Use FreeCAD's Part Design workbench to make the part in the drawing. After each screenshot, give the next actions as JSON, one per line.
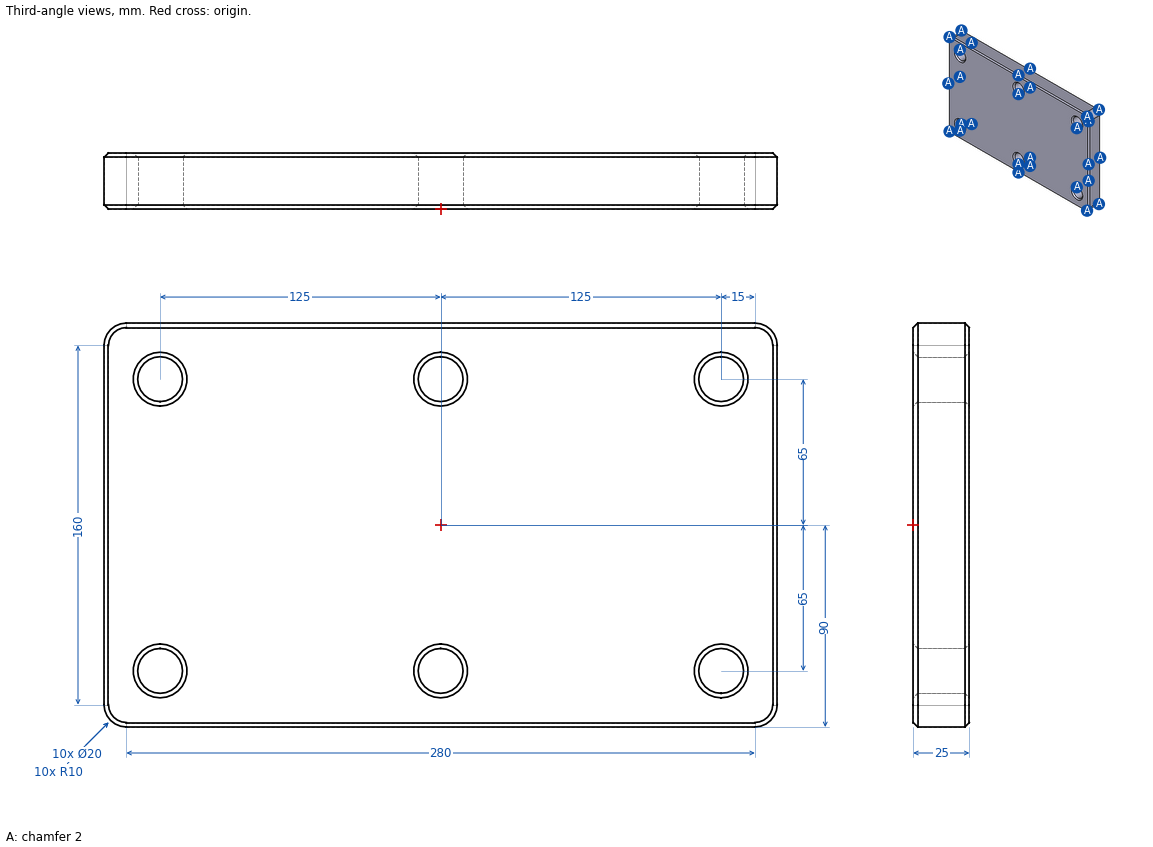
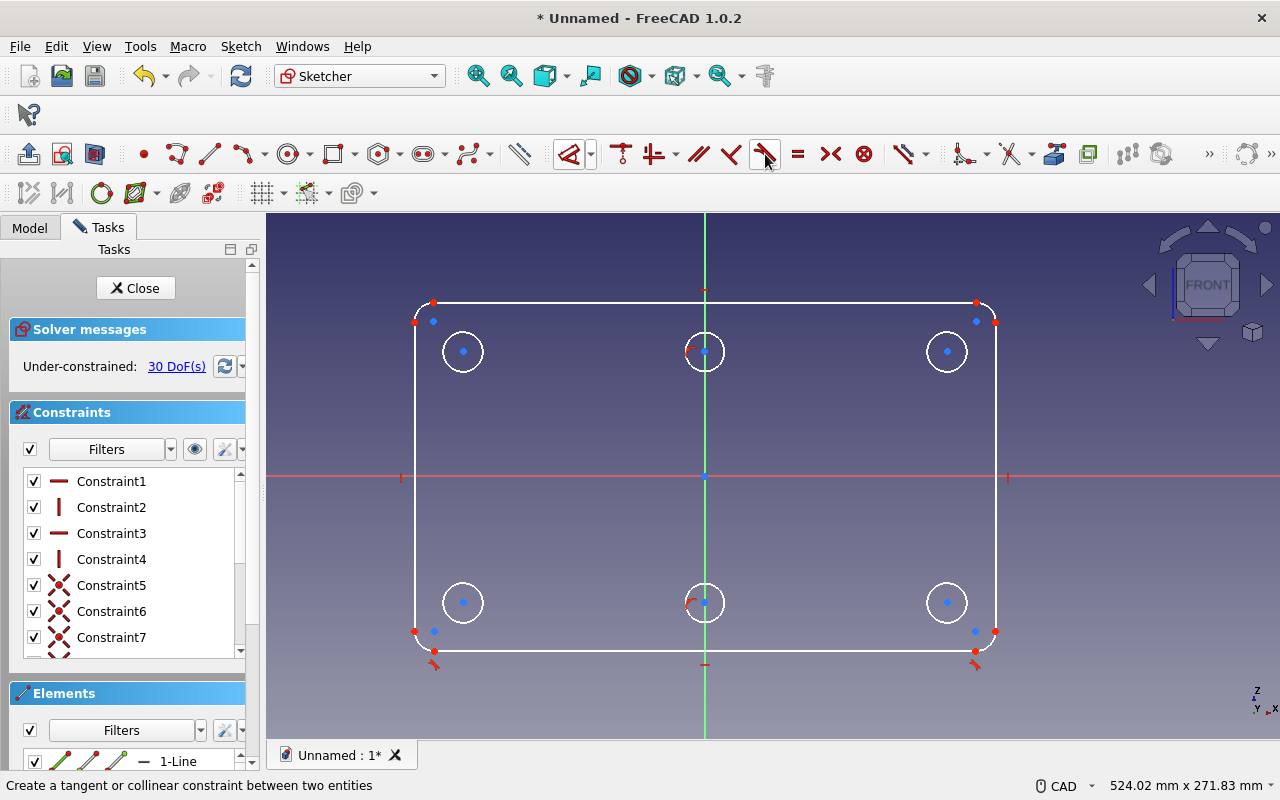
{"action": "left_click", "coordinate": [415, 539]}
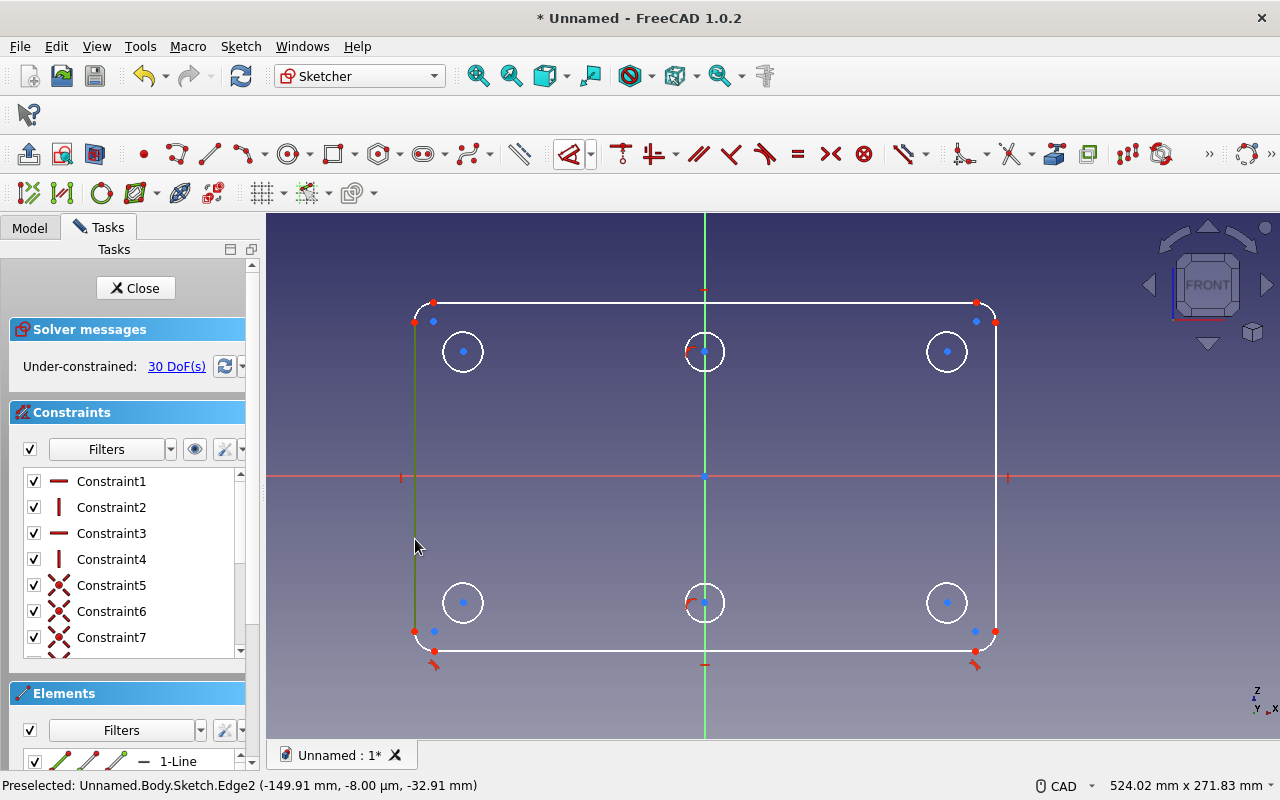
{"action": "left_click", "coordinate": [421, 645]}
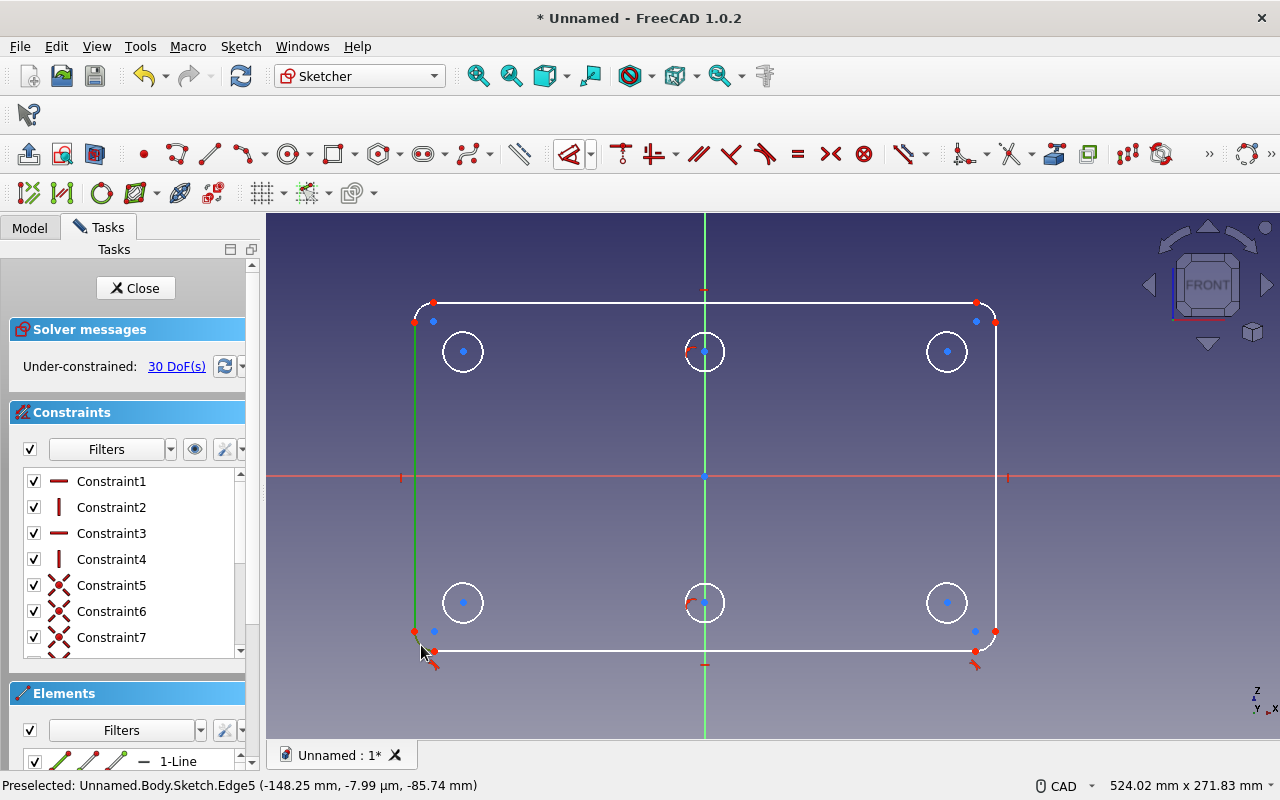
{"action": "left_click", "coordinate": [765, 154]}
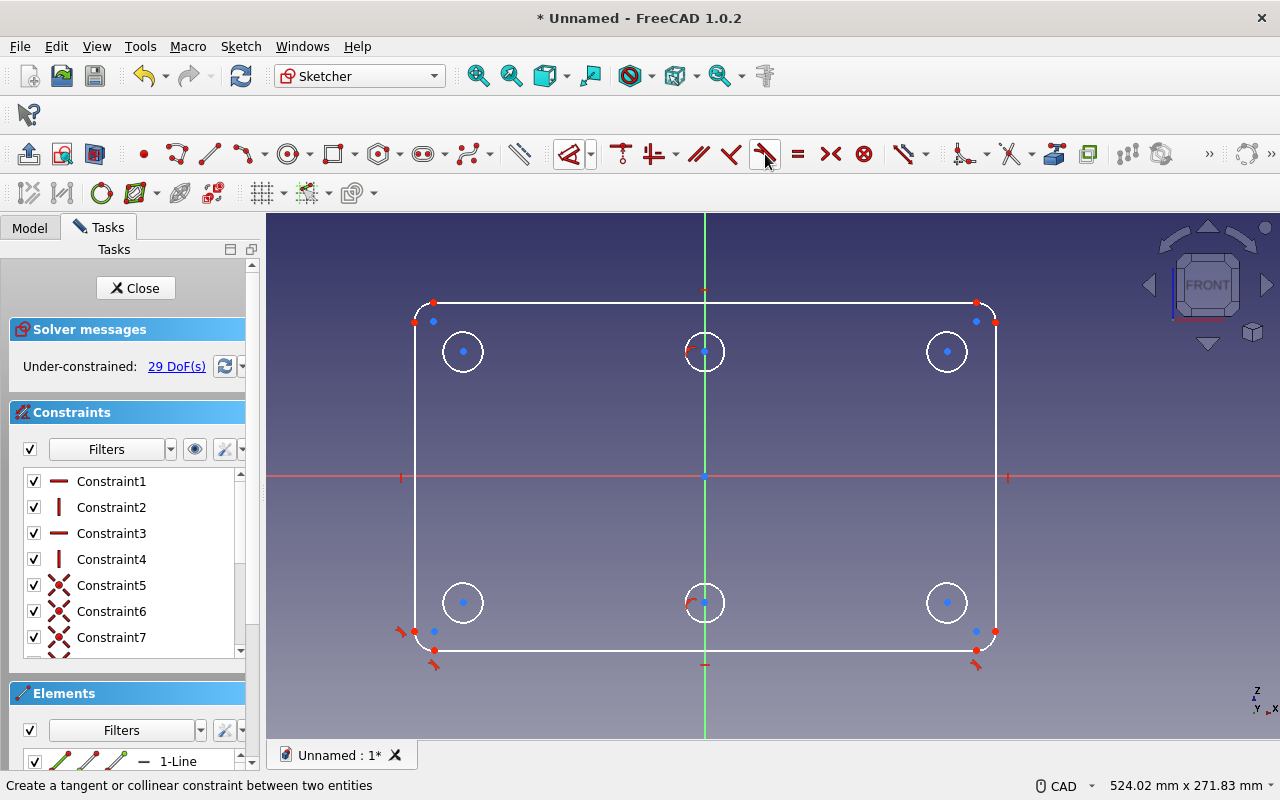
{"action": "left_click", "coordinate": [415, 539]}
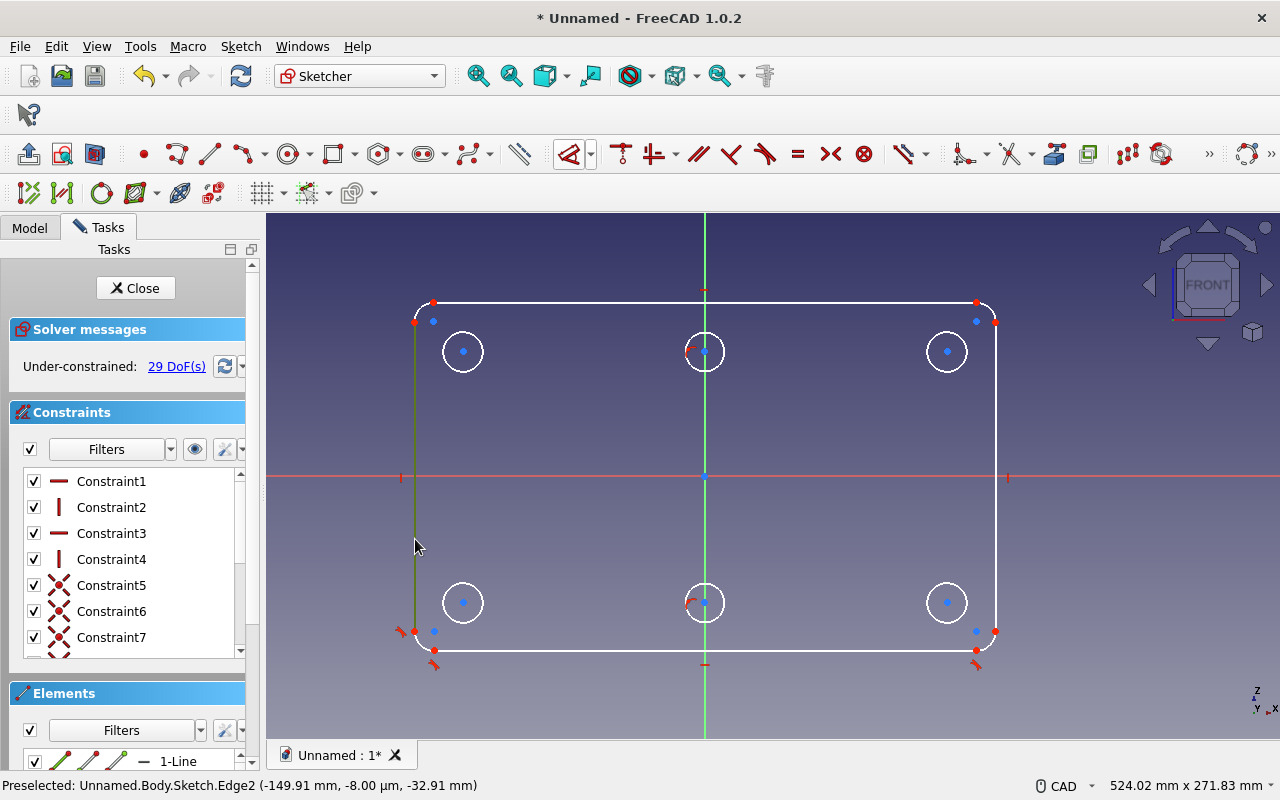
{"action": "scroll", "coordinate": [425, 305], "scroll_direction": "up", "scroll_amount": 2}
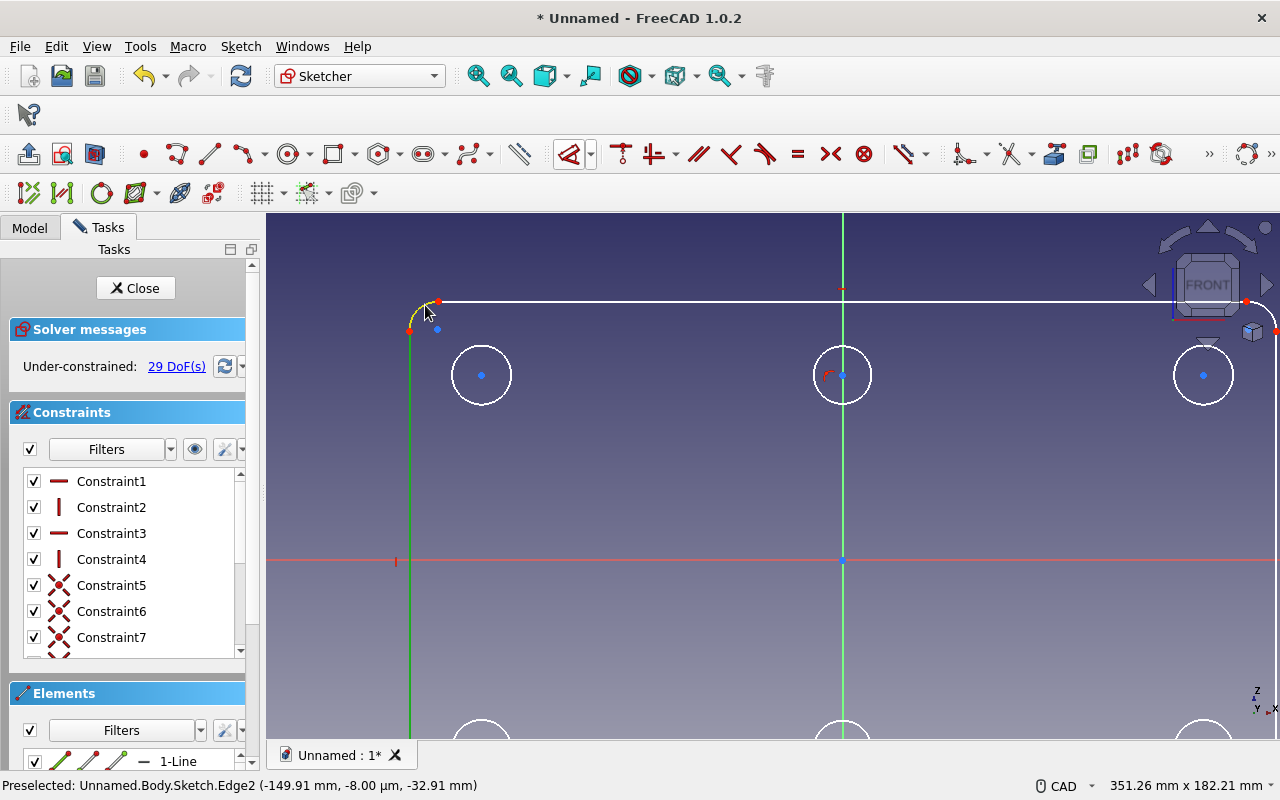
{"action": "left_click", "coordinate": [425, 305]}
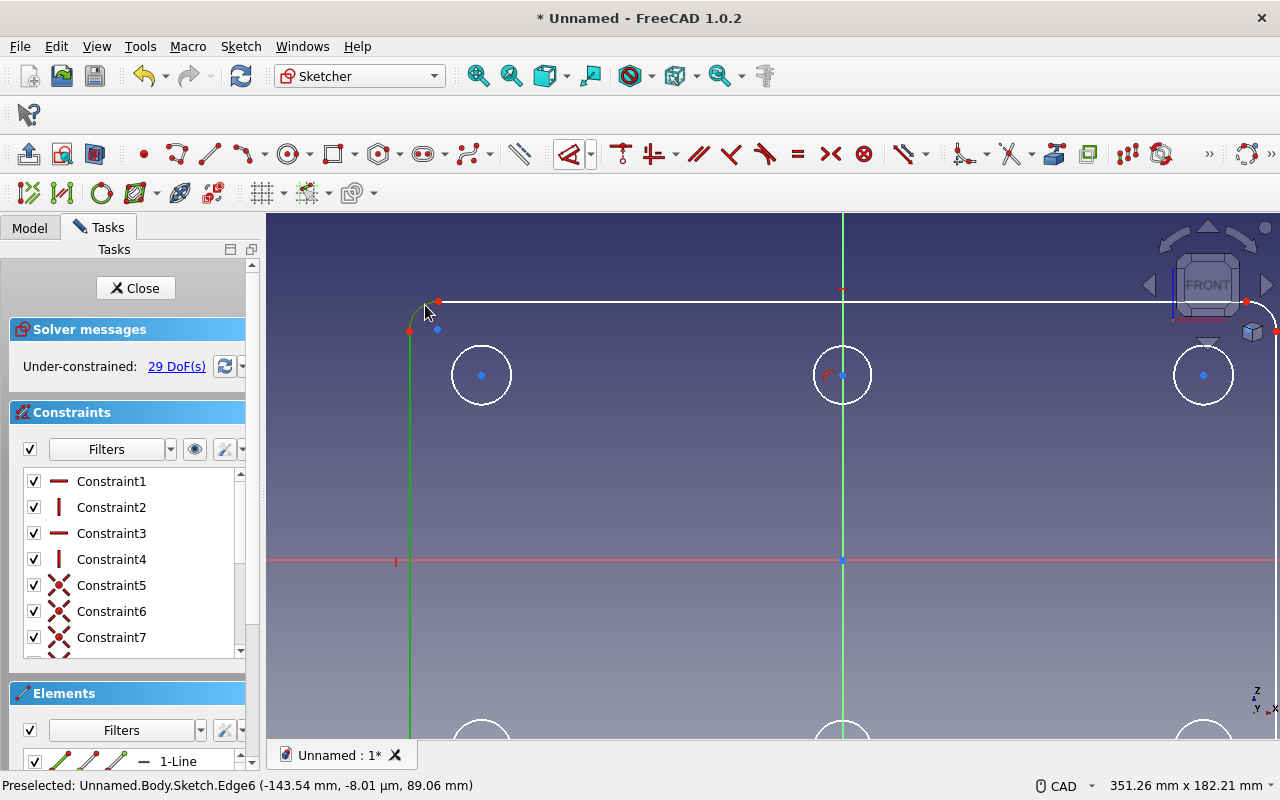
{"action": "left_click", "coordinate": [765, 154]}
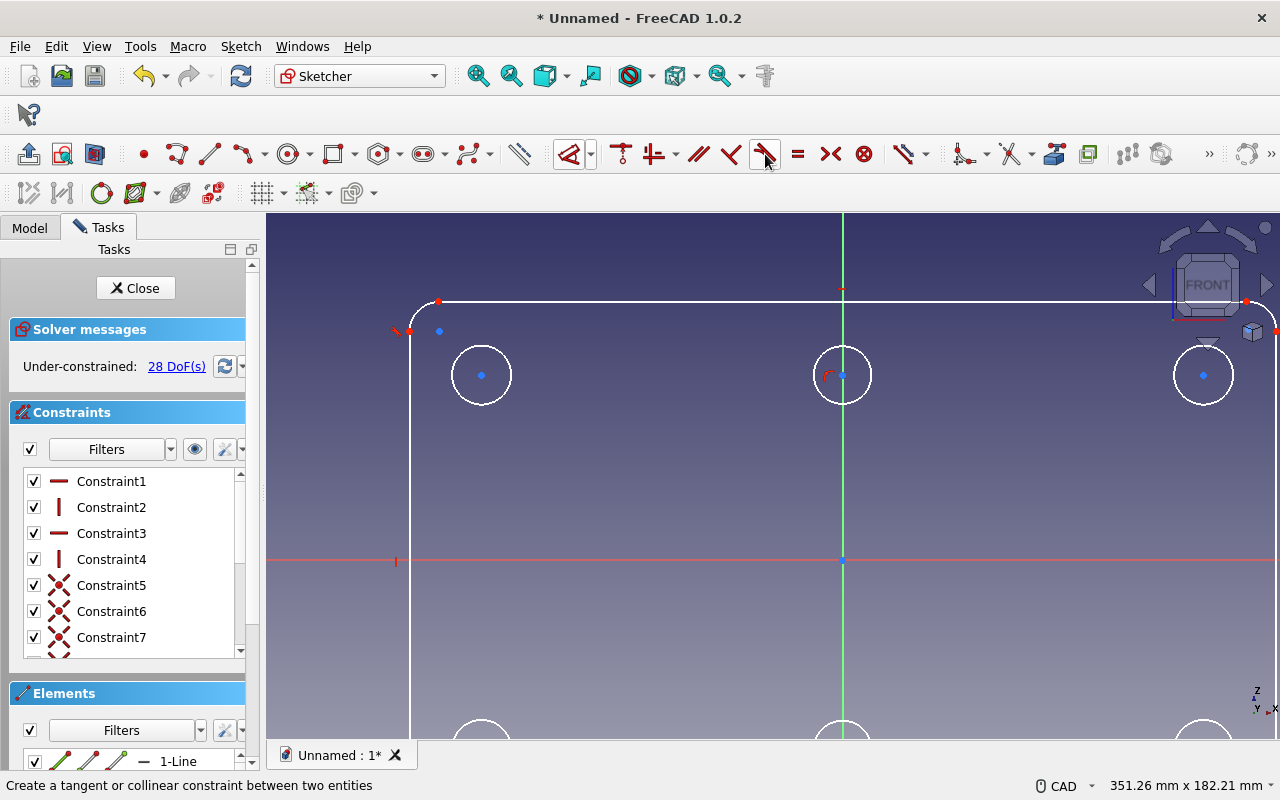
{"action": "left_click", "coordinate": [681, 302]}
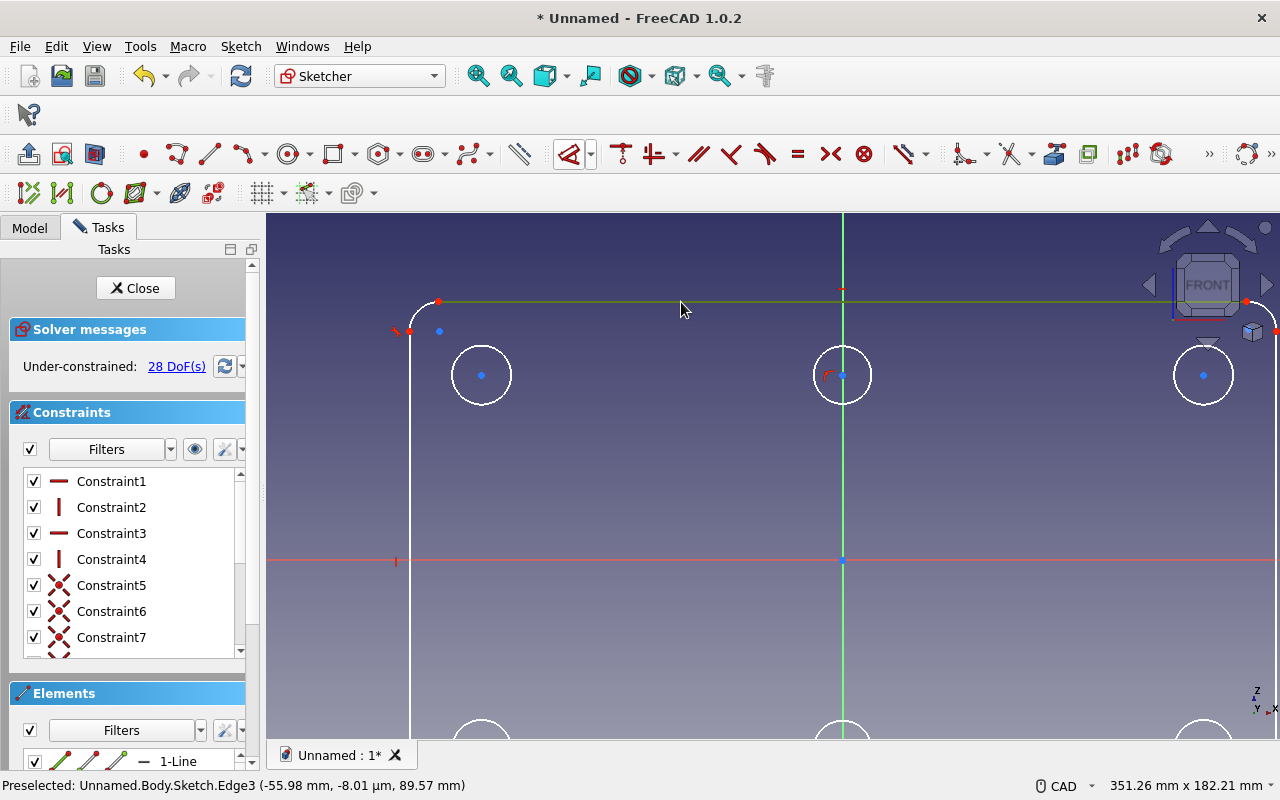
{"action": "left_click", "coordinate": [425, 306]}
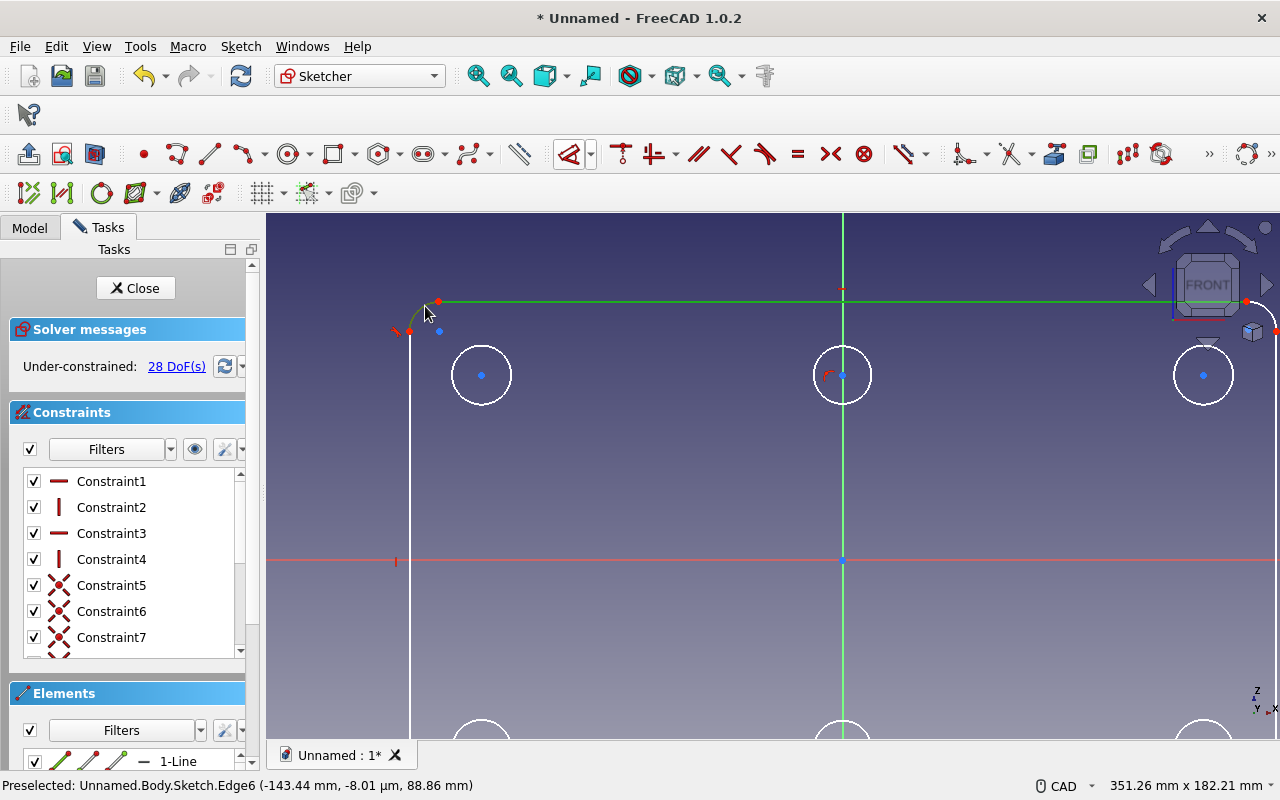
{"action": "left_click", "coordinate": [765, 154]}